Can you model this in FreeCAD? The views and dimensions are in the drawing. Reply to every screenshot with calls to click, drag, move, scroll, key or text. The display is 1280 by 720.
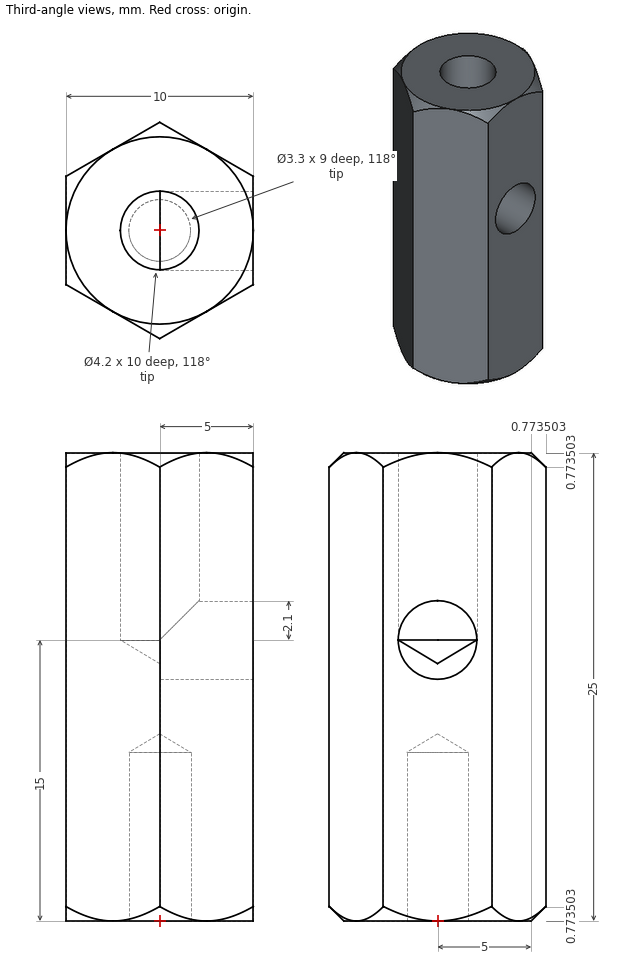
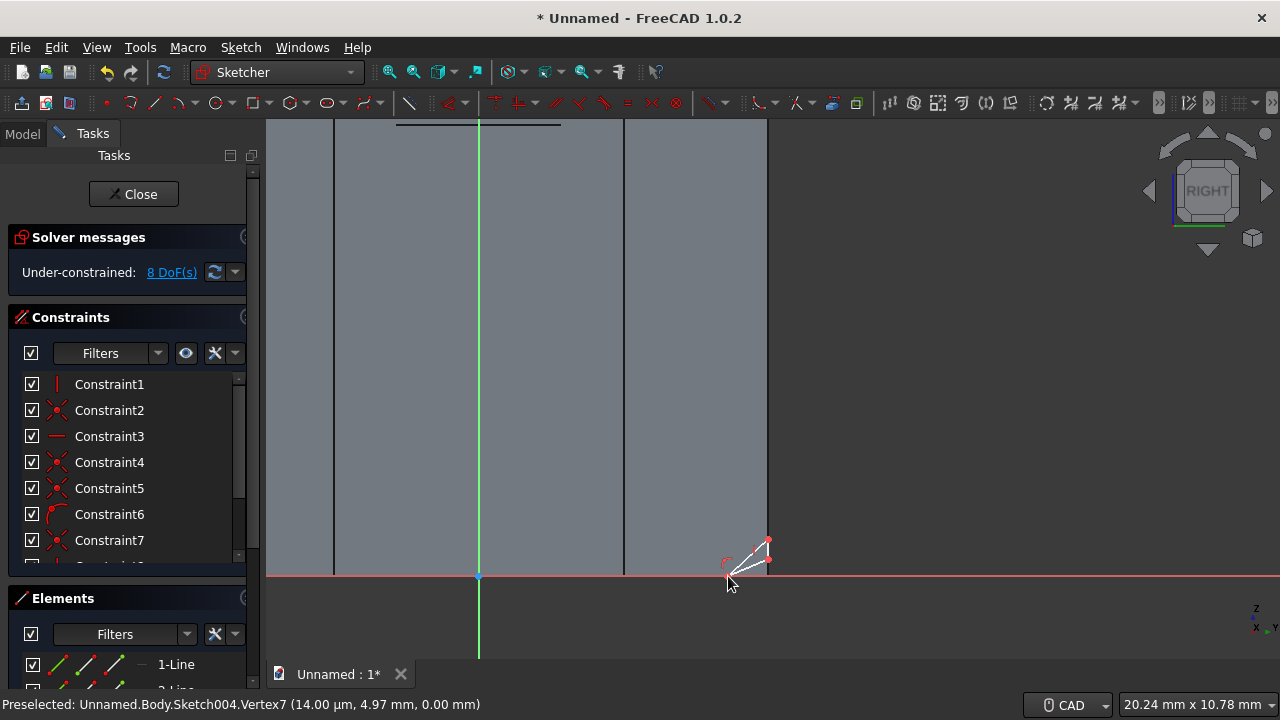
scroll(756, 564, up, 2)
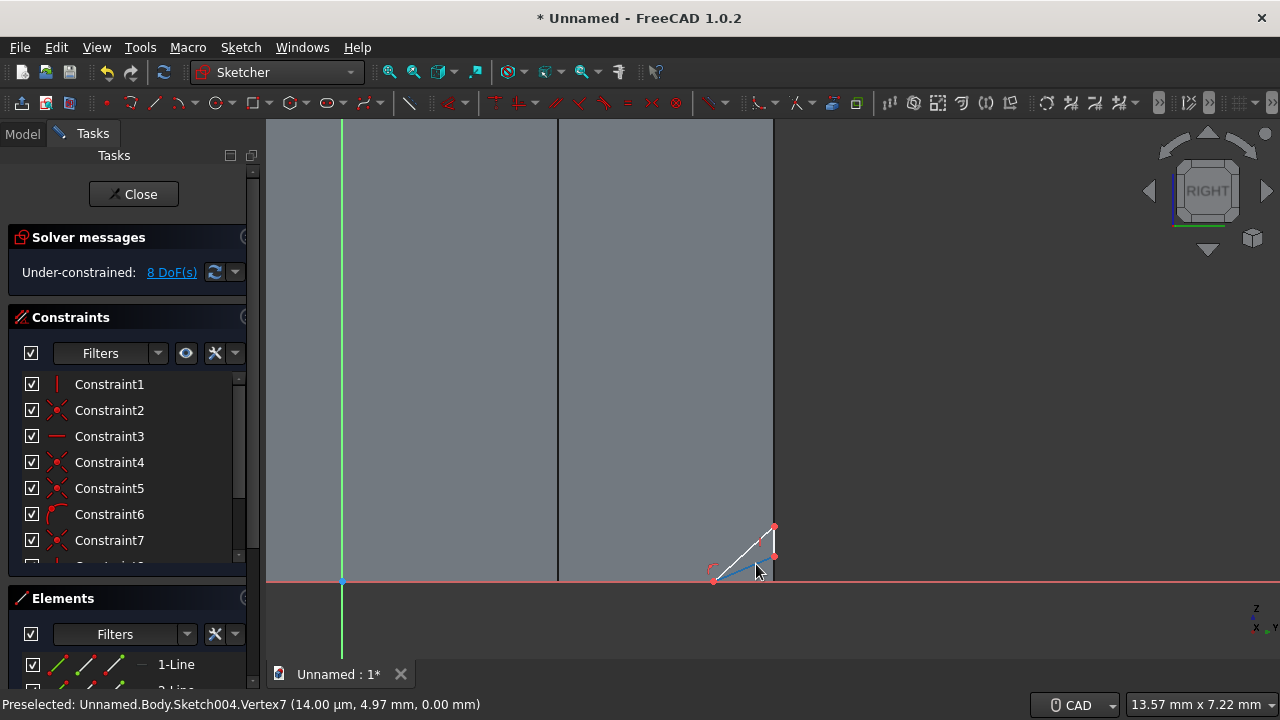
click(756, 564)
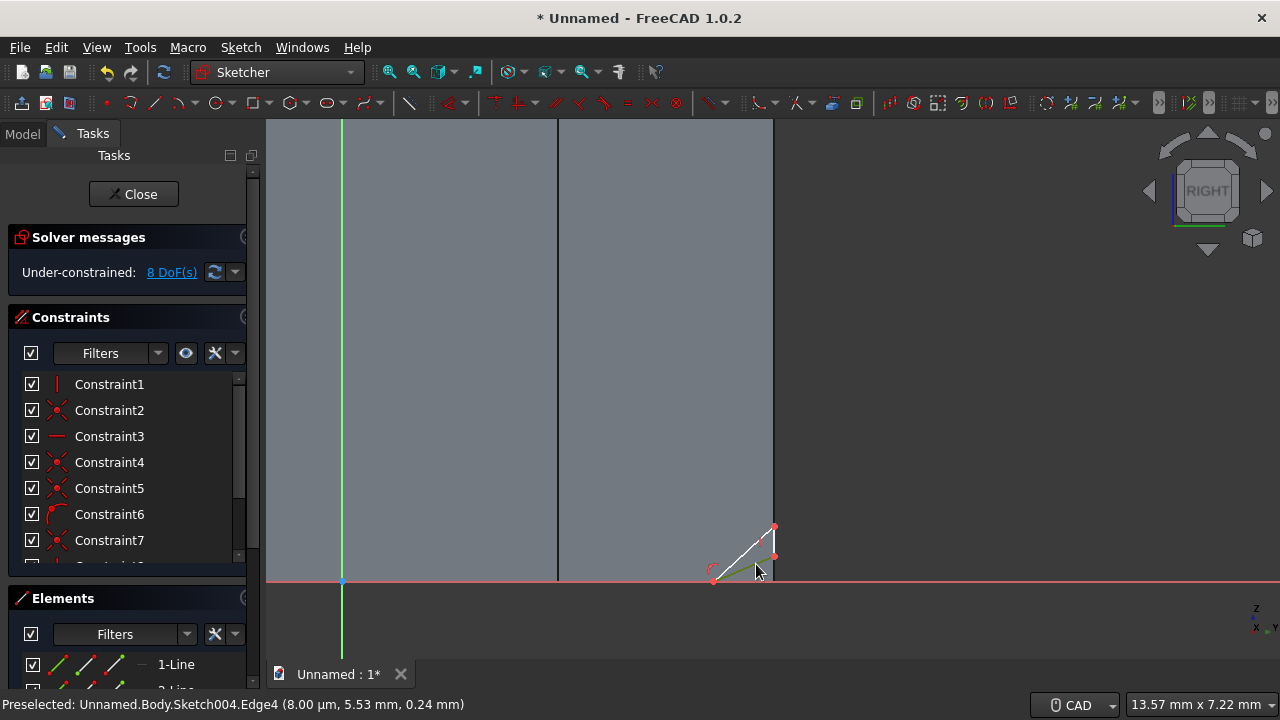
click(538, 104)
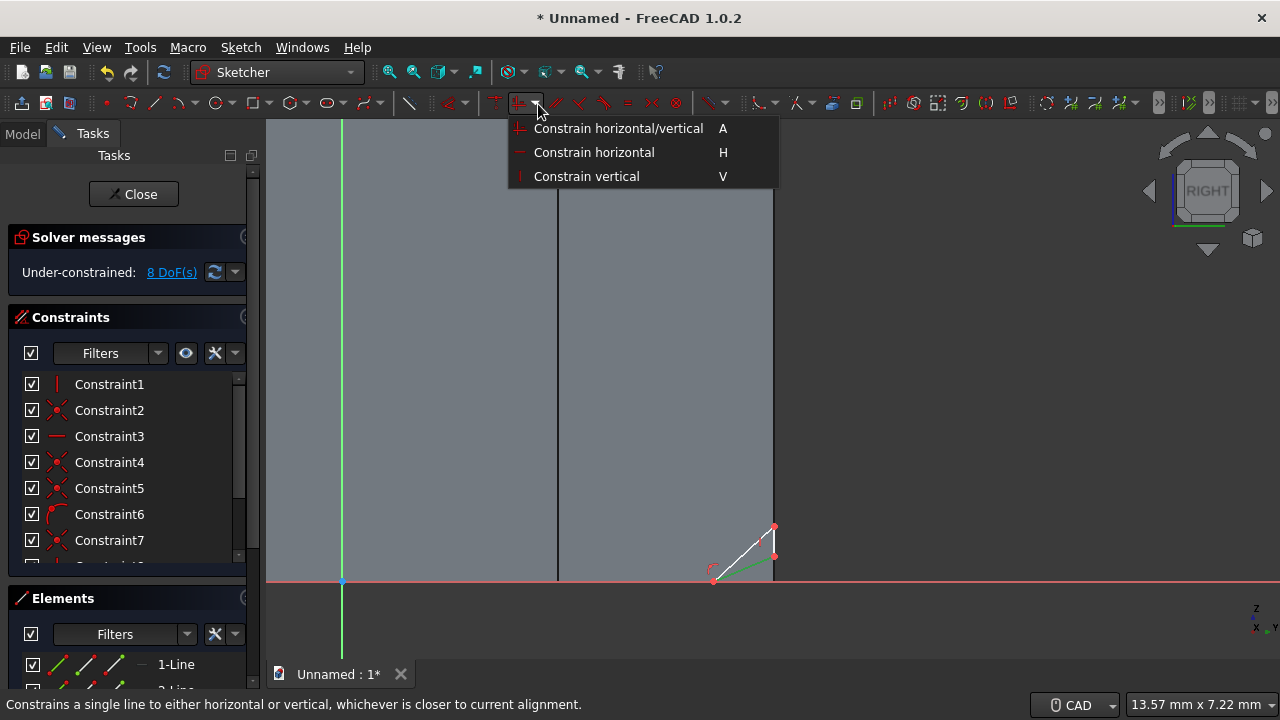
click(644, 152)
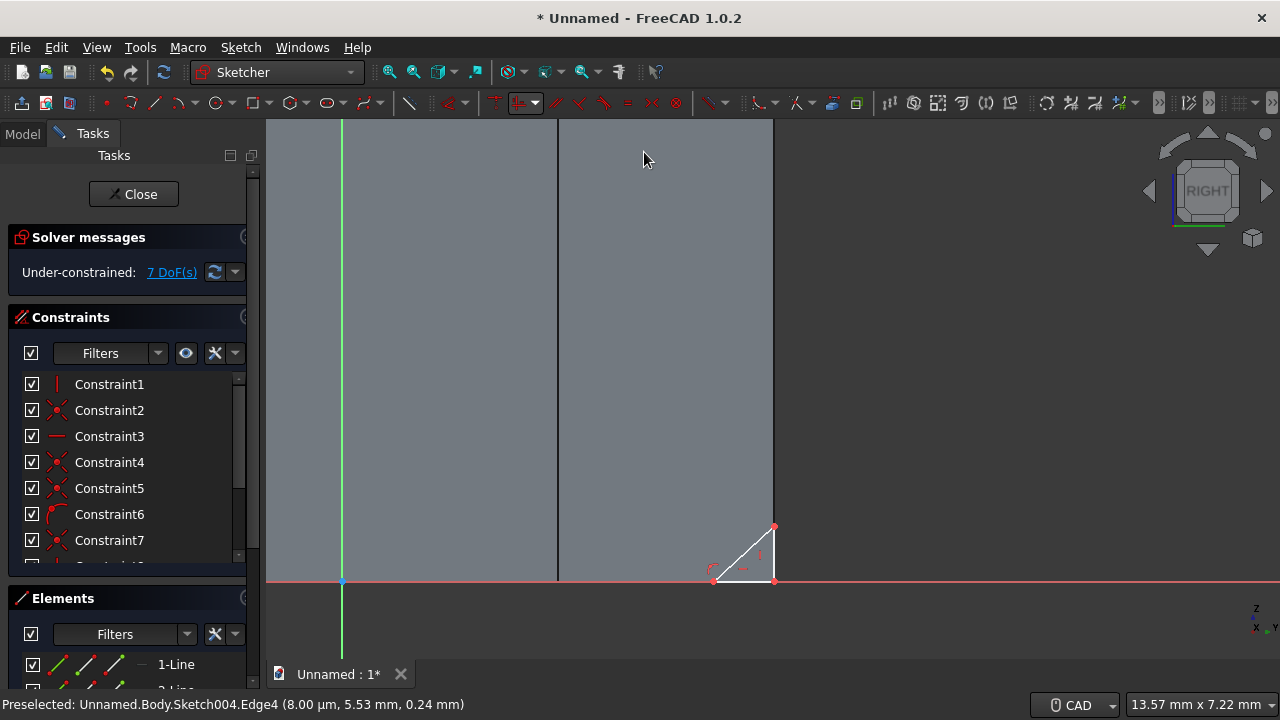
click(448, 104)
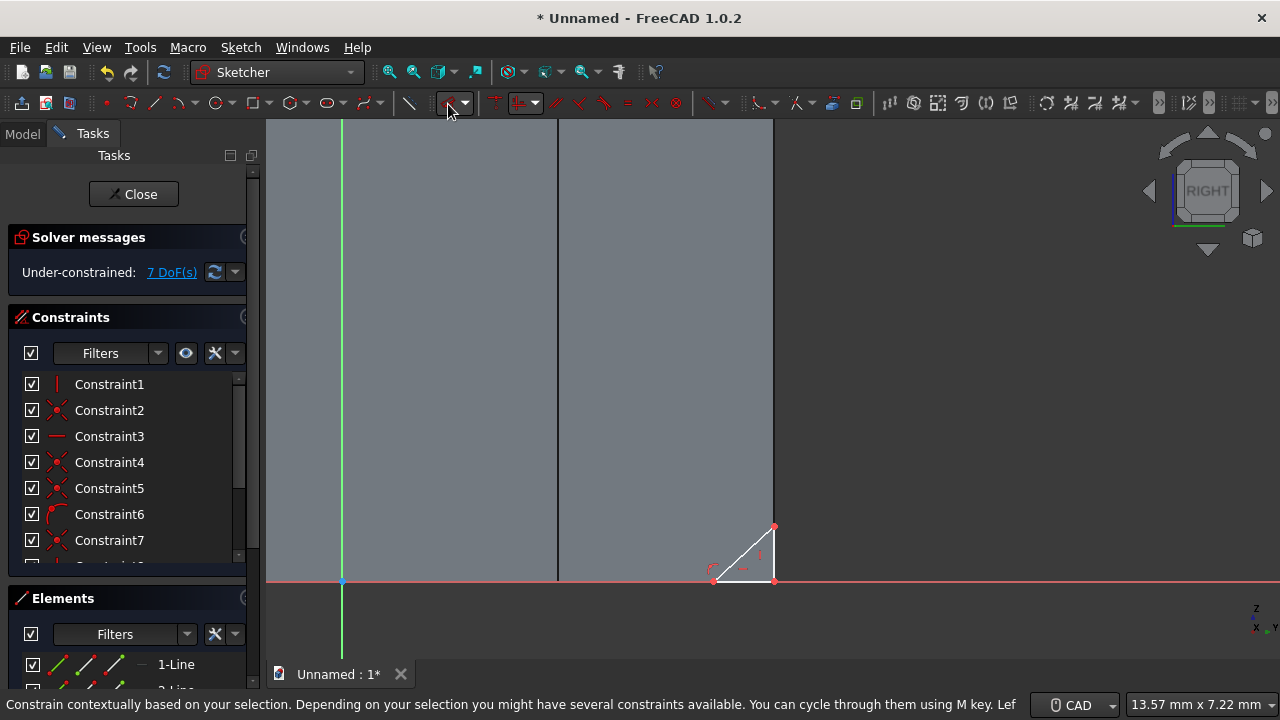
scroll(742, 577, down, 8)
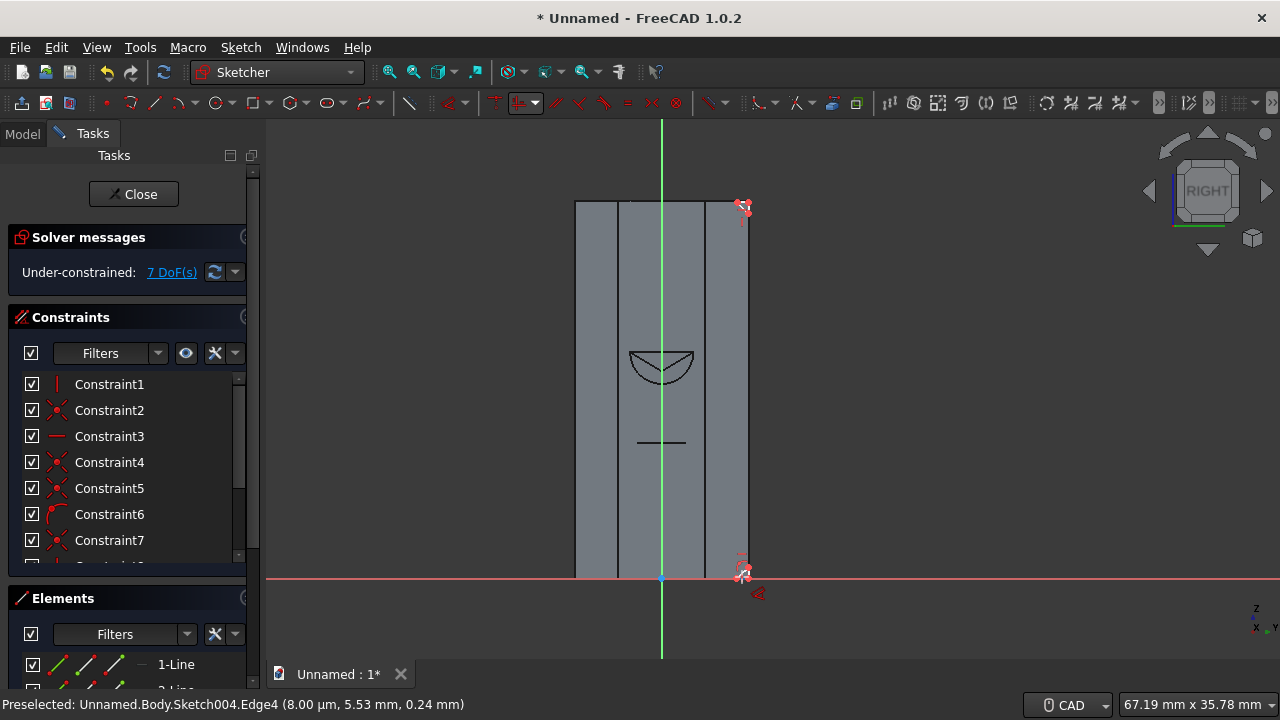
click(737, 202)
click(699, 613)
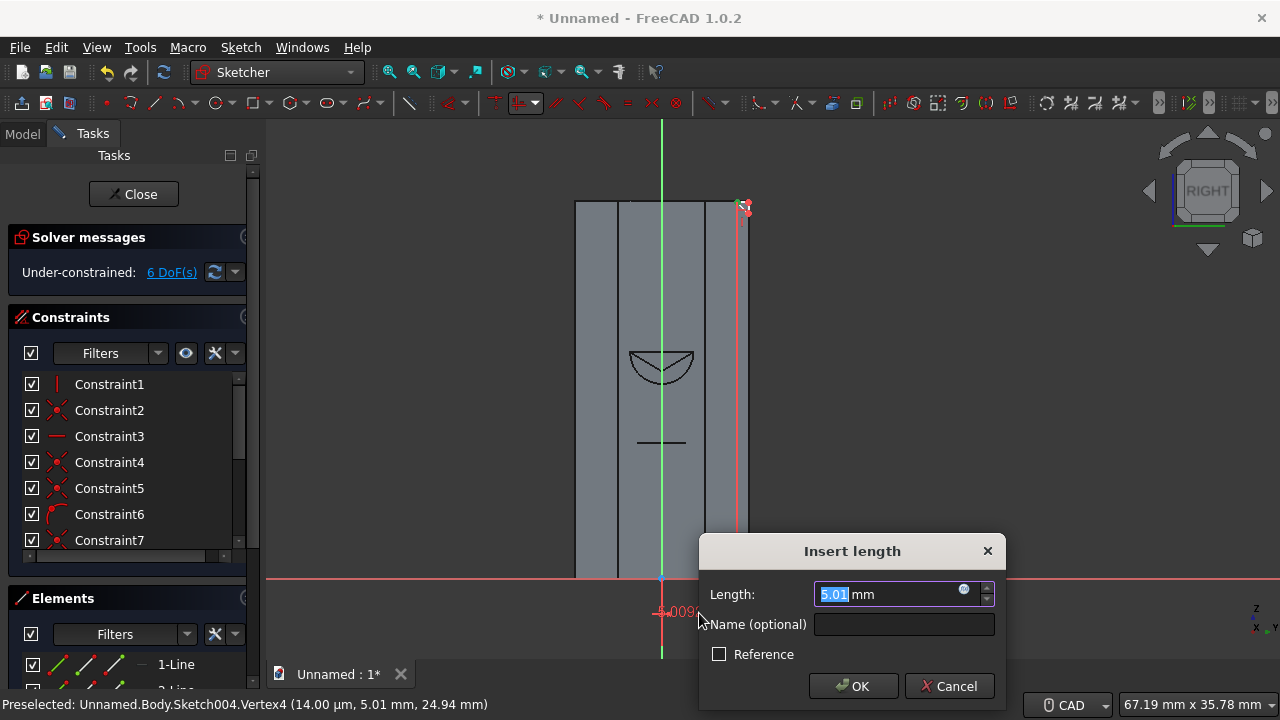
text(5)
key(Return)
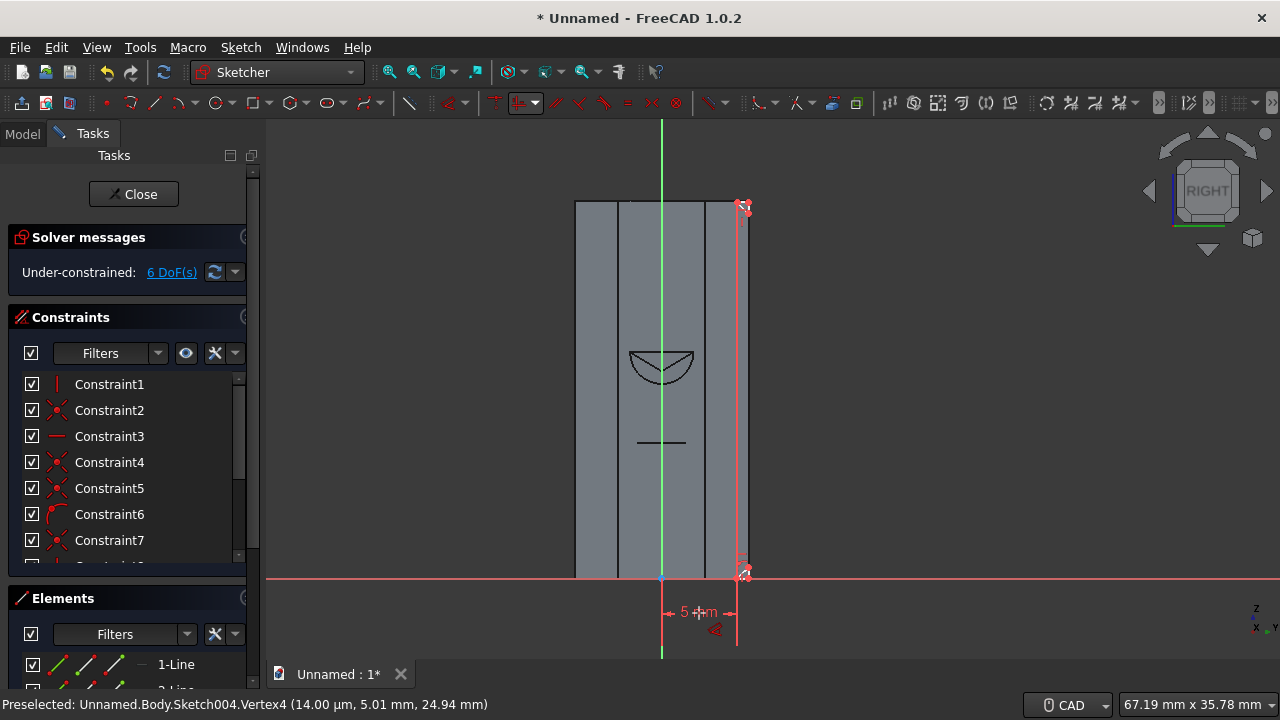
click(737, 579)
click(699, 545)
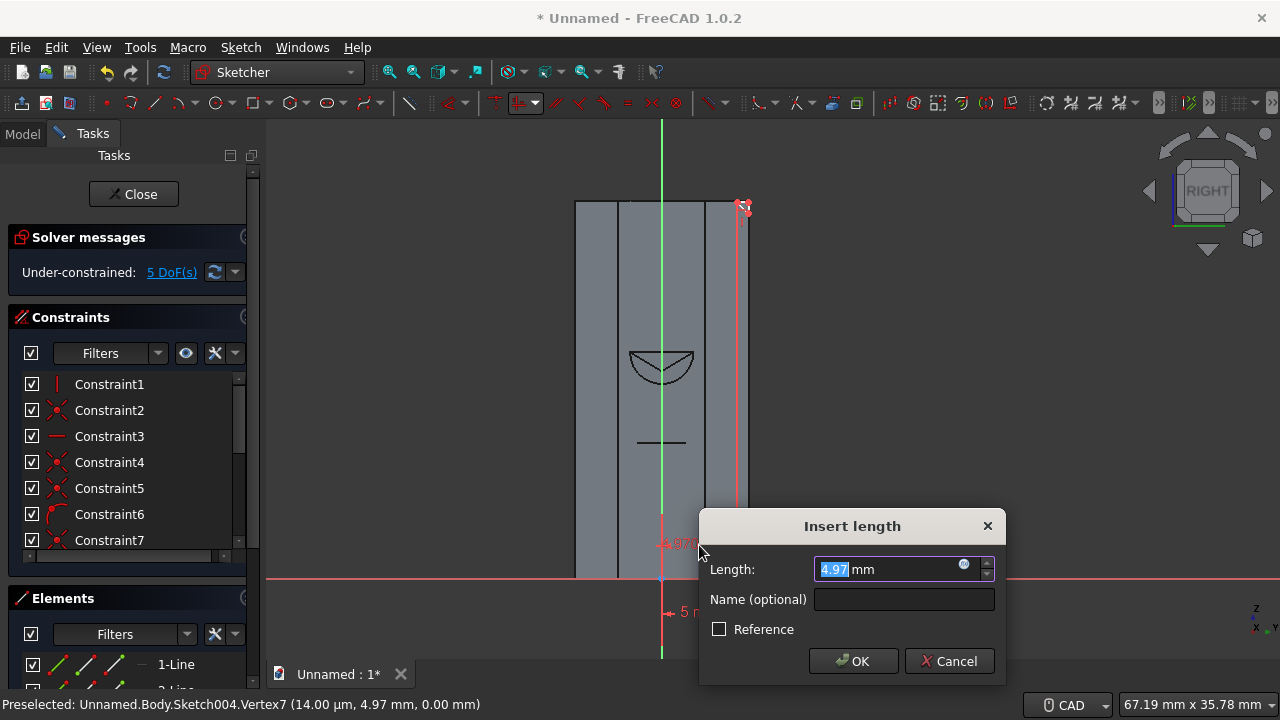
text(5)
key(Return)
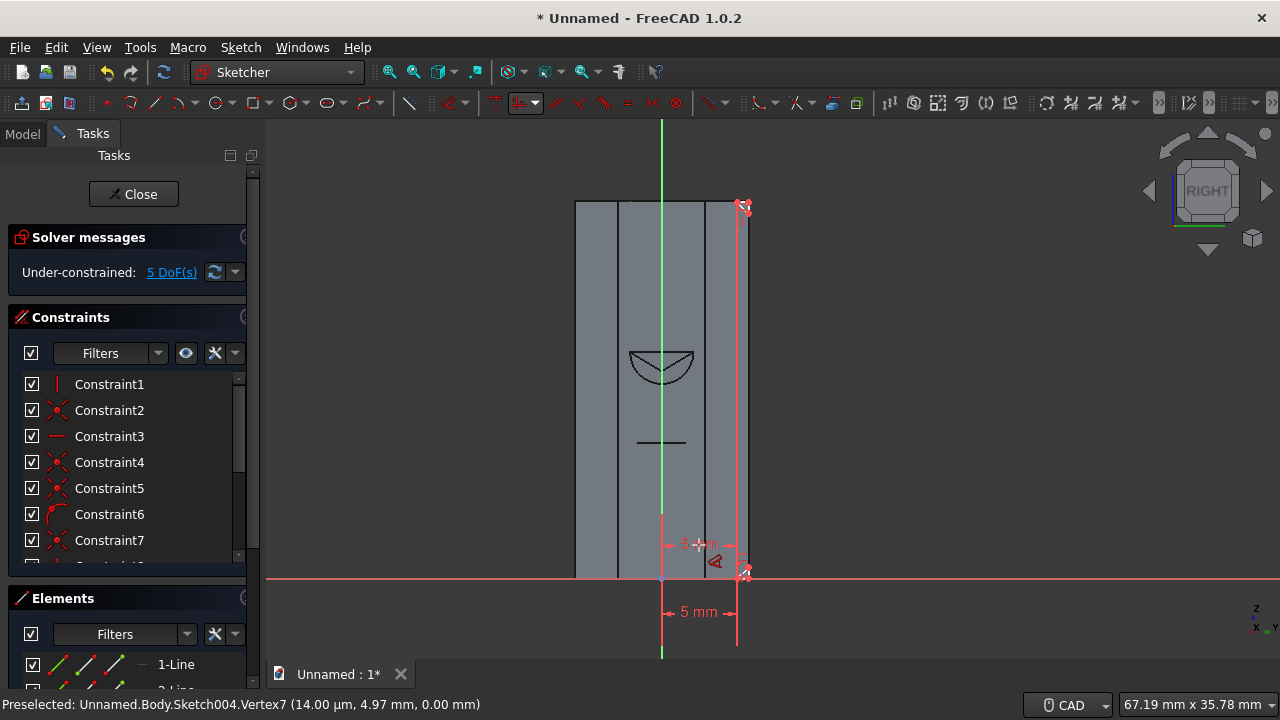
click(749, 202)
click(628, 390)